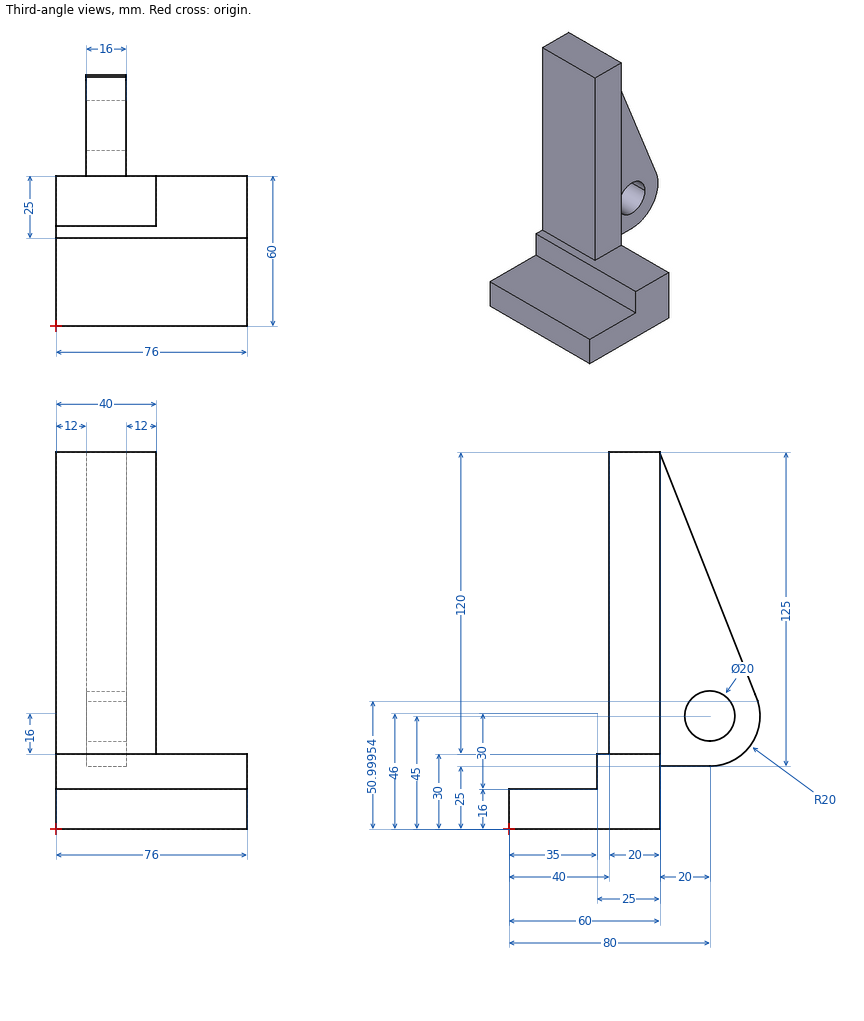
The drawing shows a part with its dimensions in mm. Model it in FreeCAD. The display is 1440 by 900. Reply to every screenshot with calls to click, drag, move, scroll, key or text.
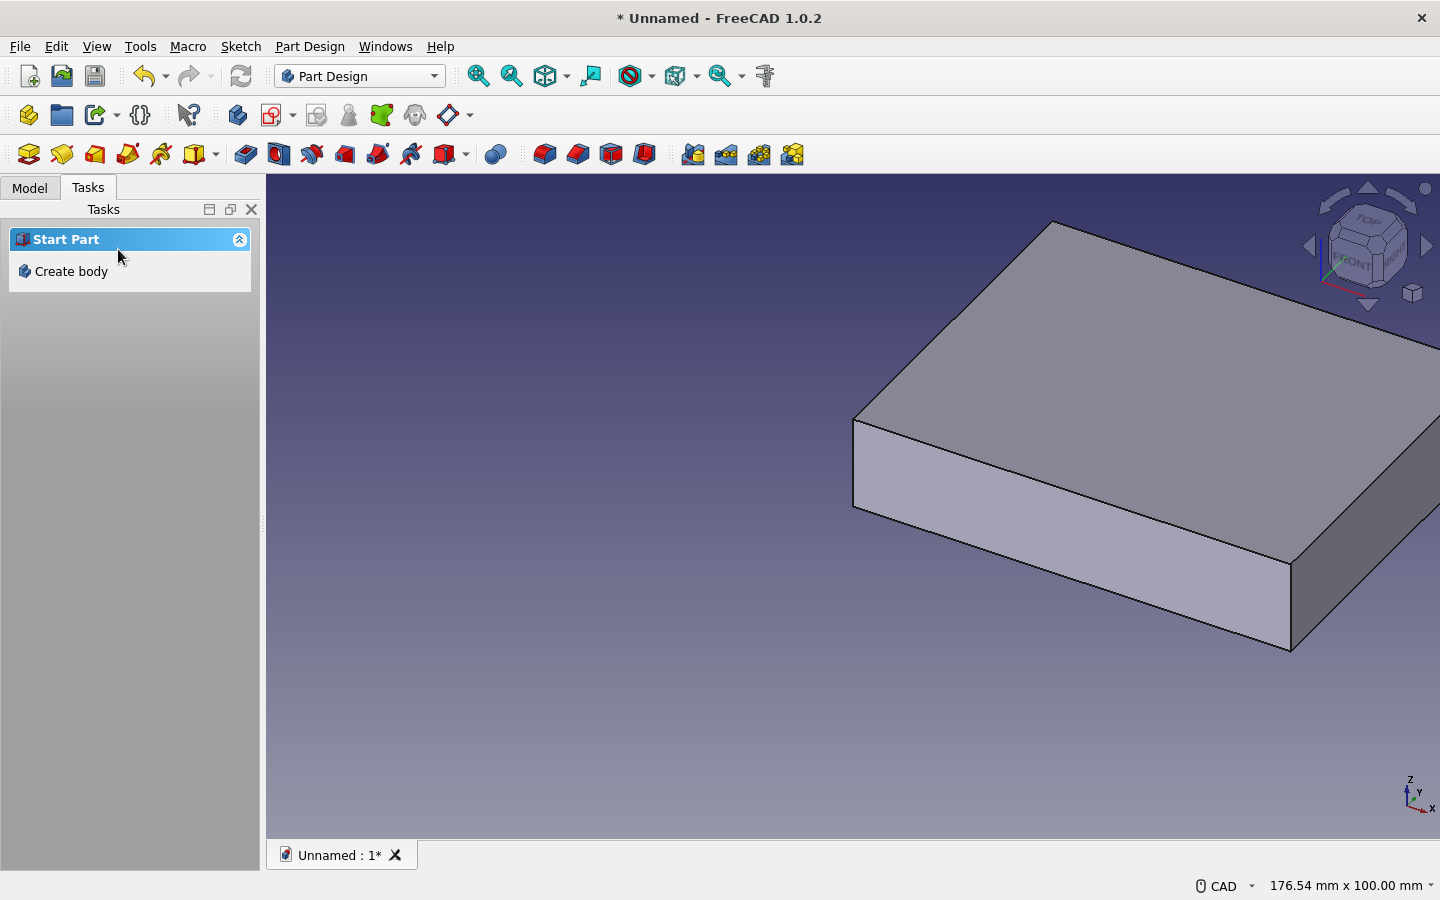
key(v)
key(f)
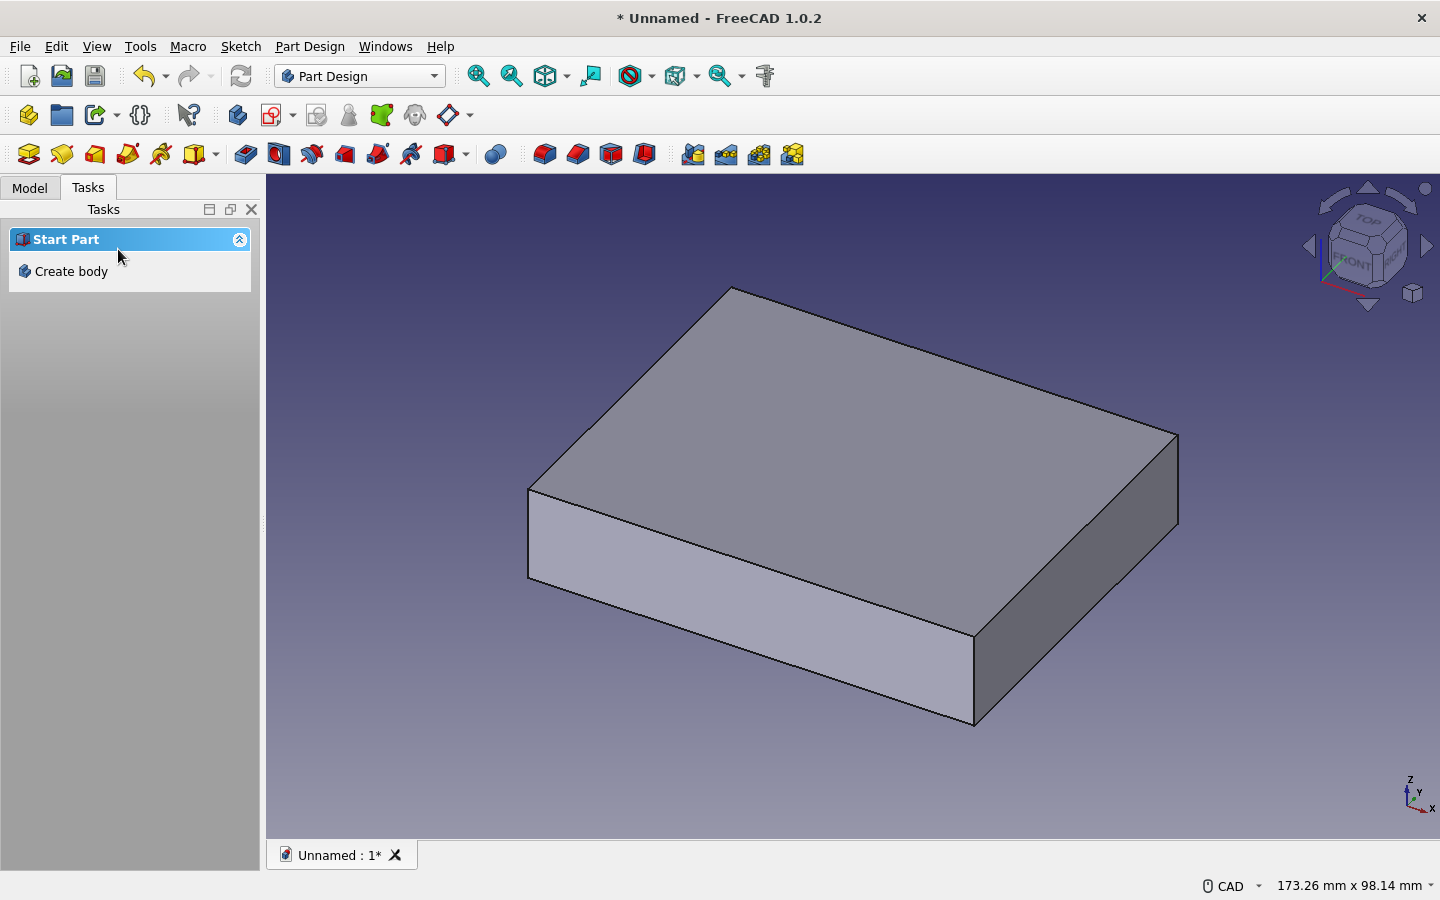
click(1134, 522)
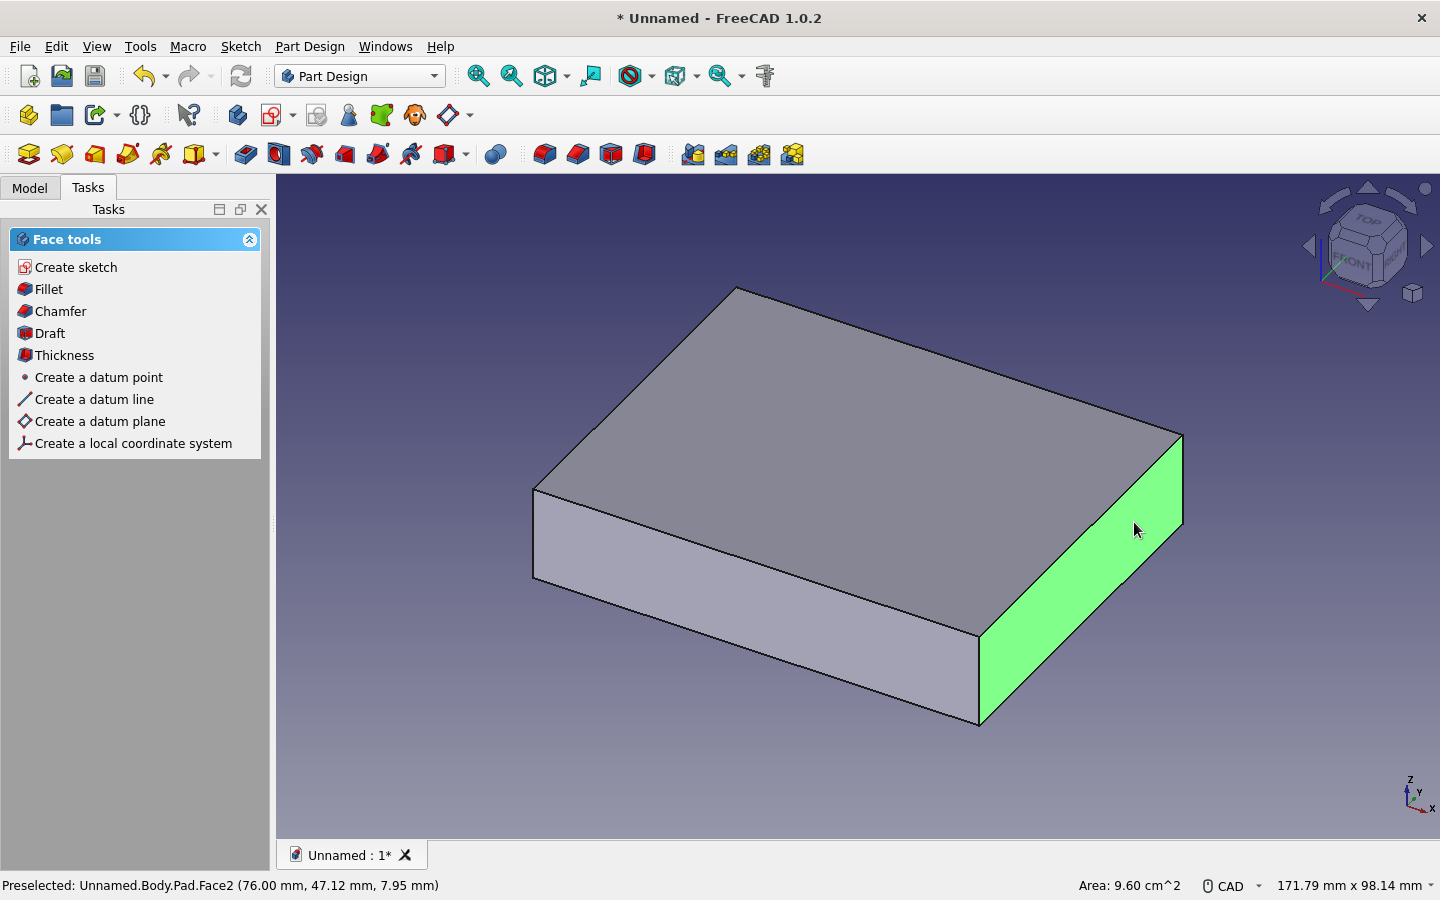
click(270, 116)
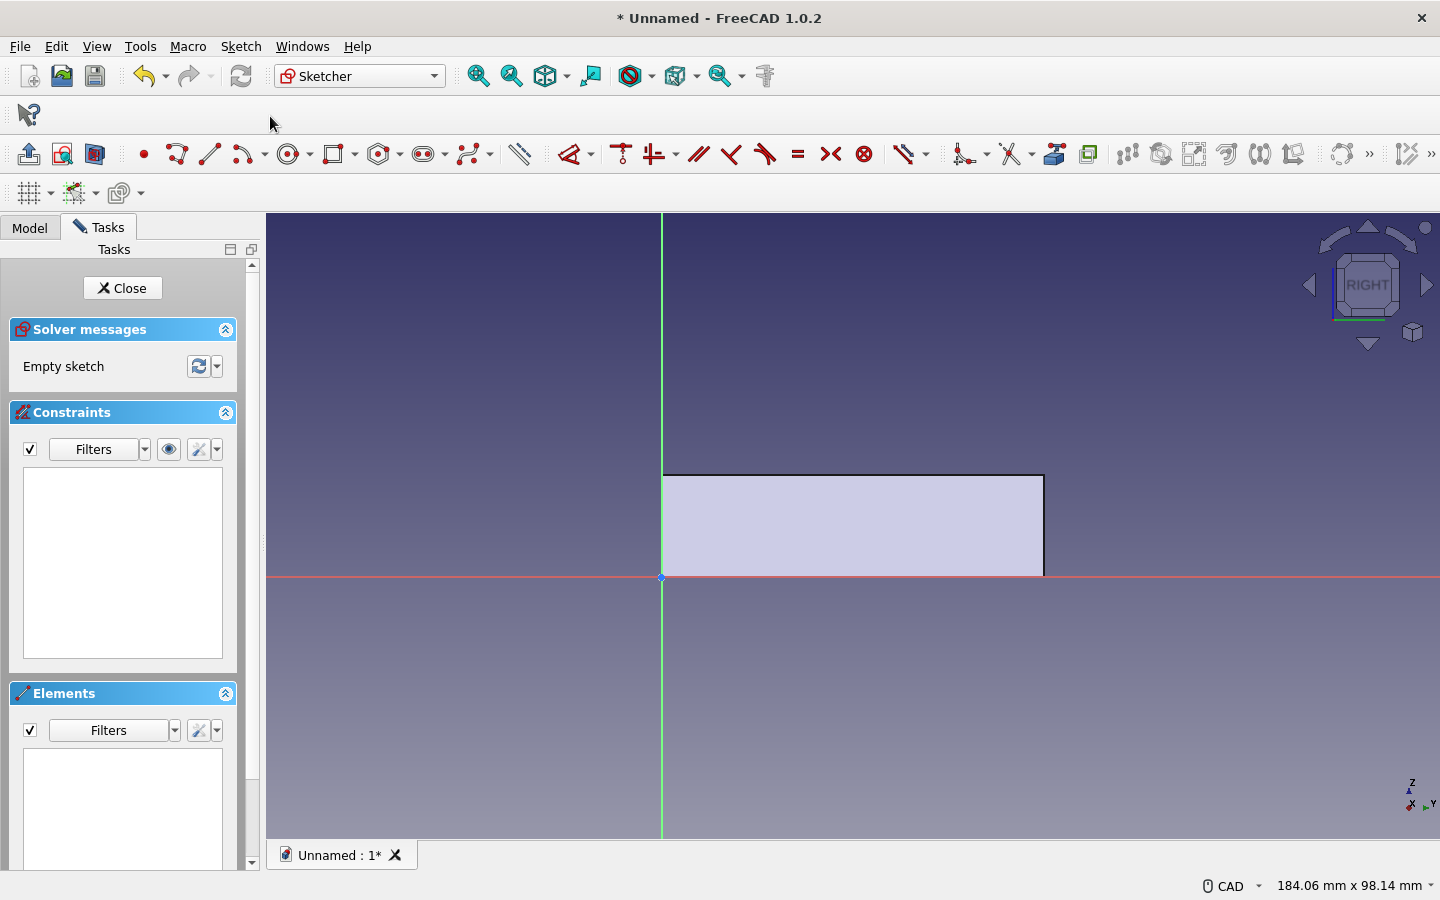
scroll(992, 241, up, 2)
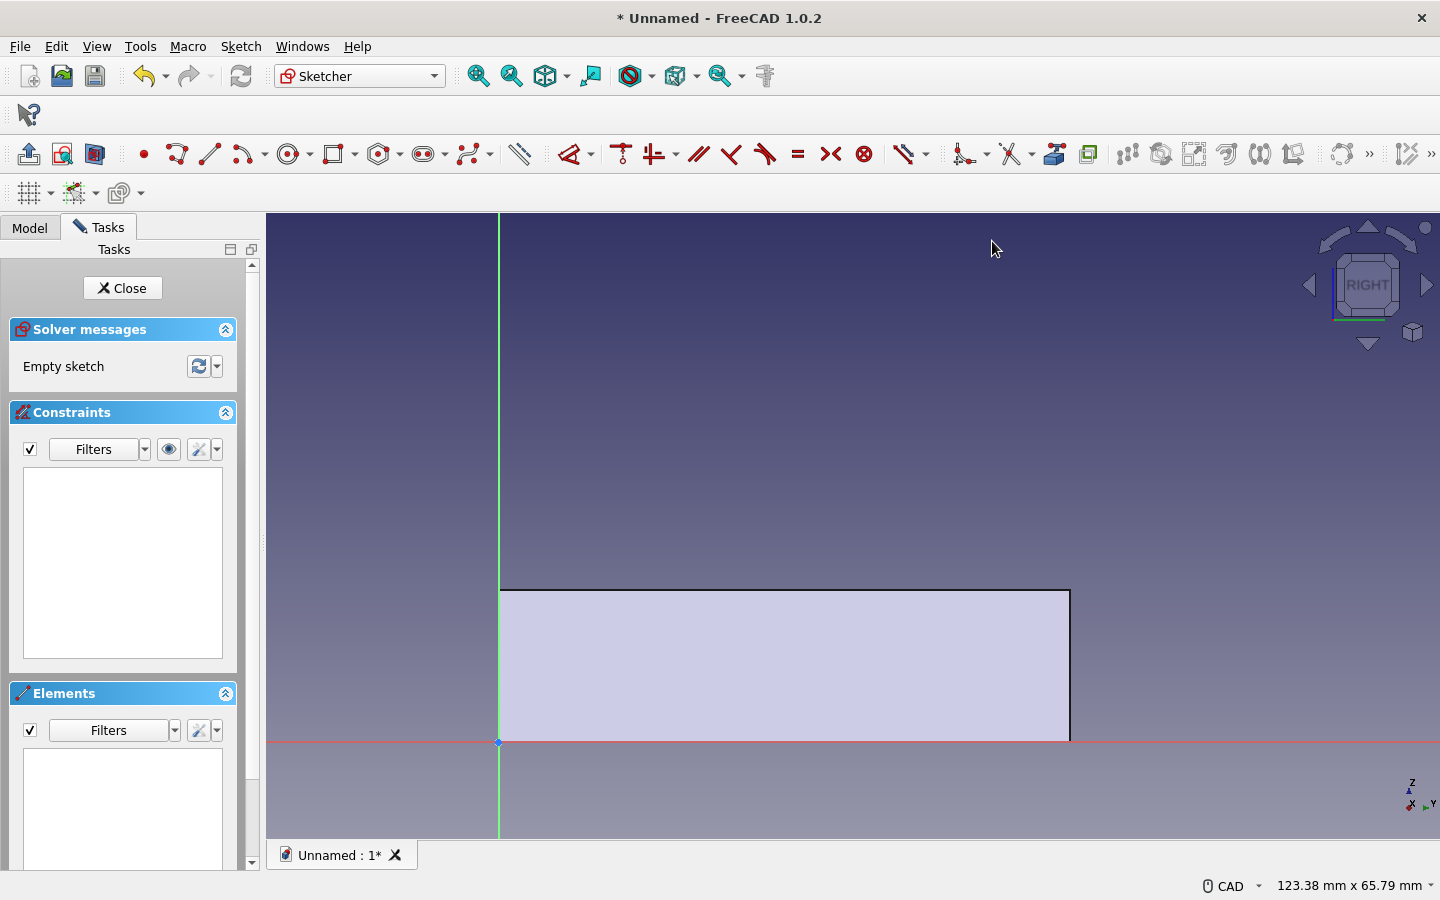
key(g)
key(r)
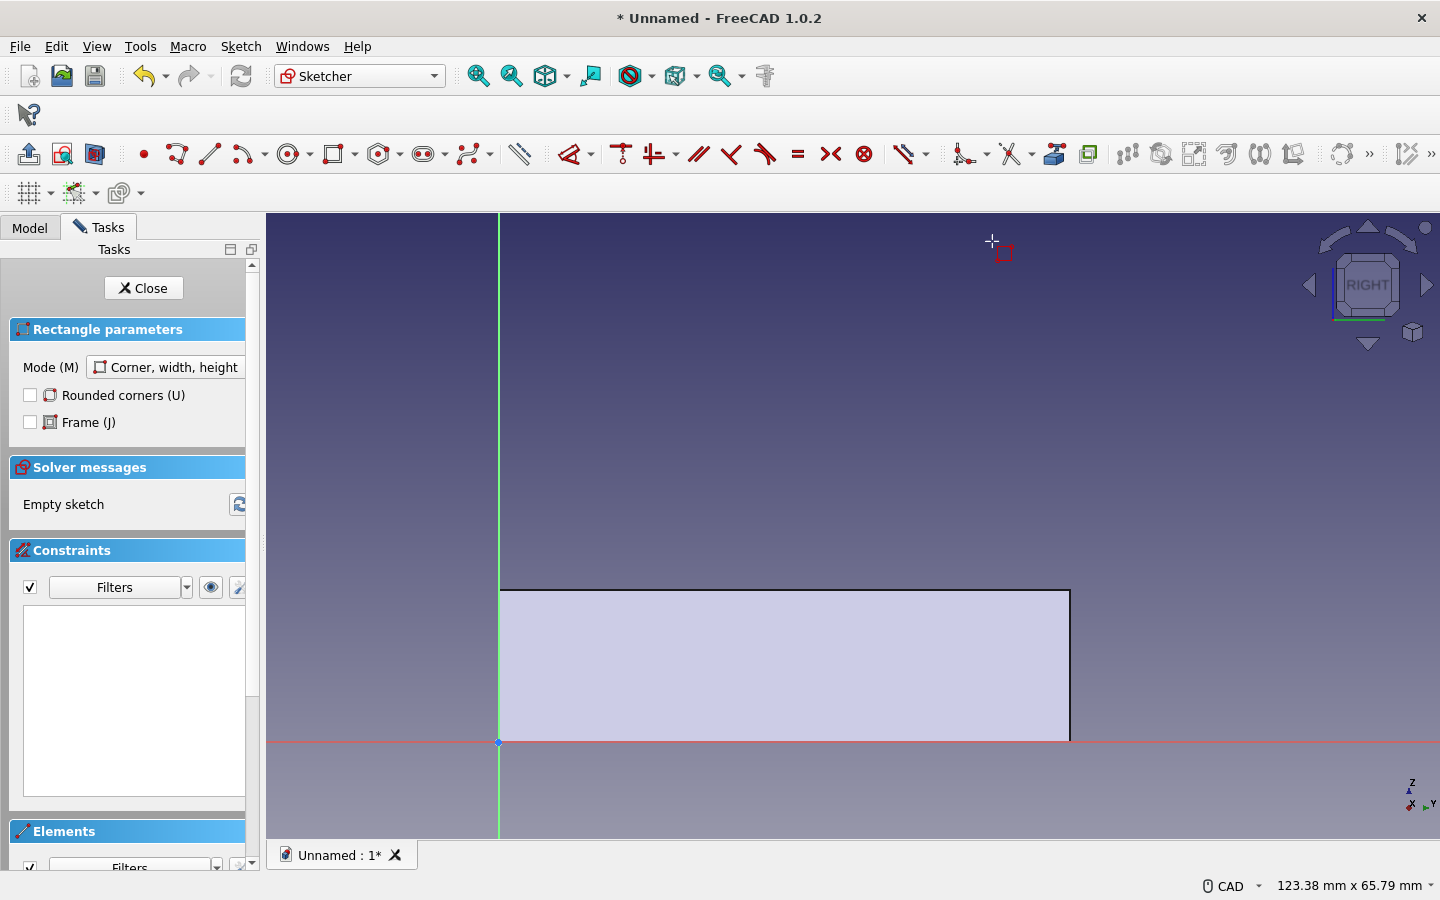
click(832, 305)
click(1070, 590)
key(Escape)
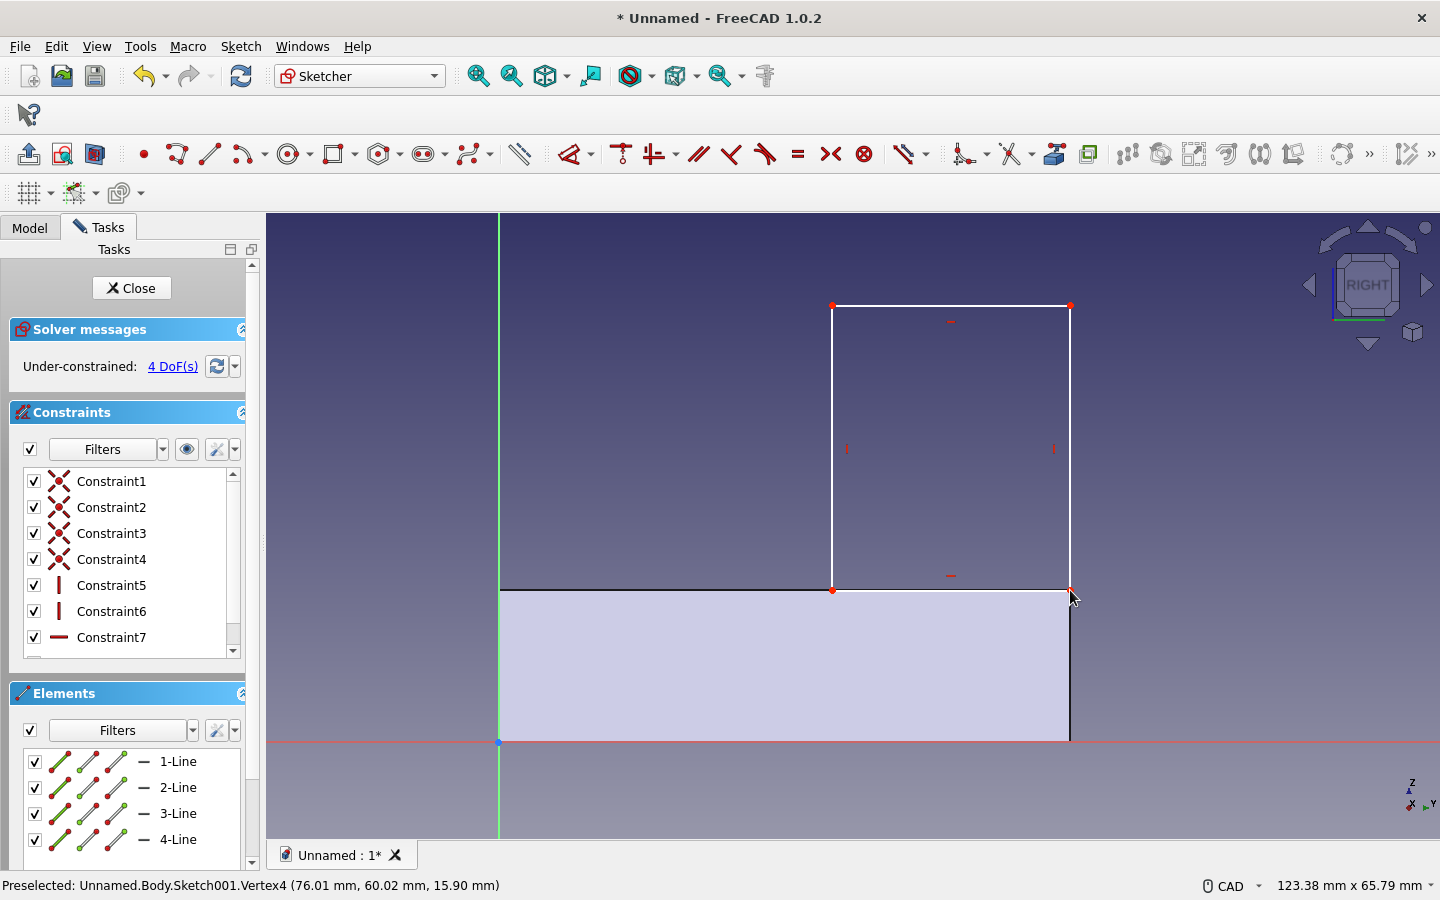
click(568, 154)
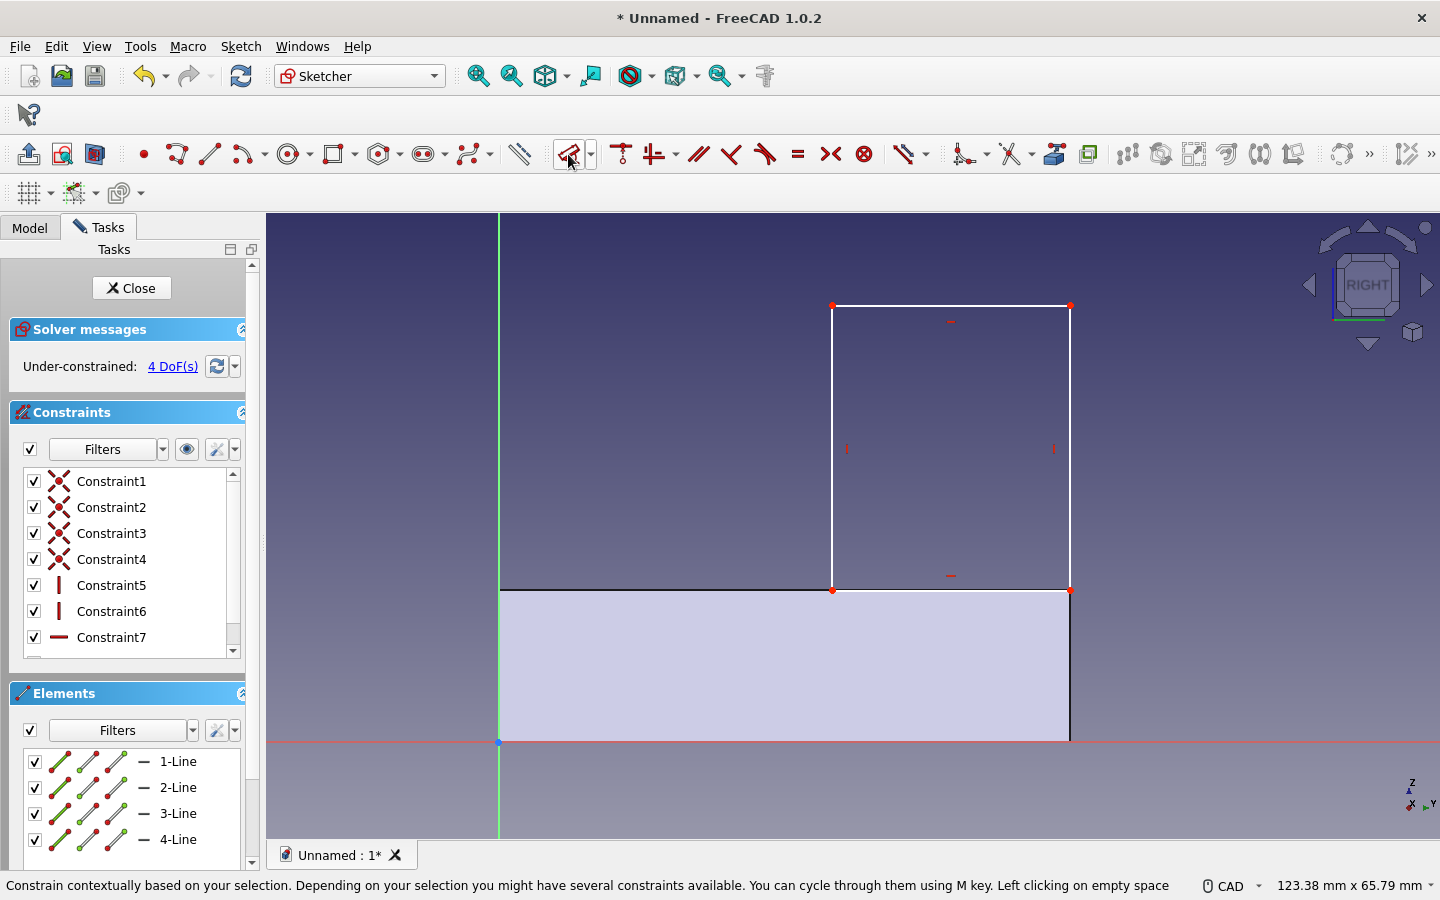
click(832, 391)
click(866, 448)